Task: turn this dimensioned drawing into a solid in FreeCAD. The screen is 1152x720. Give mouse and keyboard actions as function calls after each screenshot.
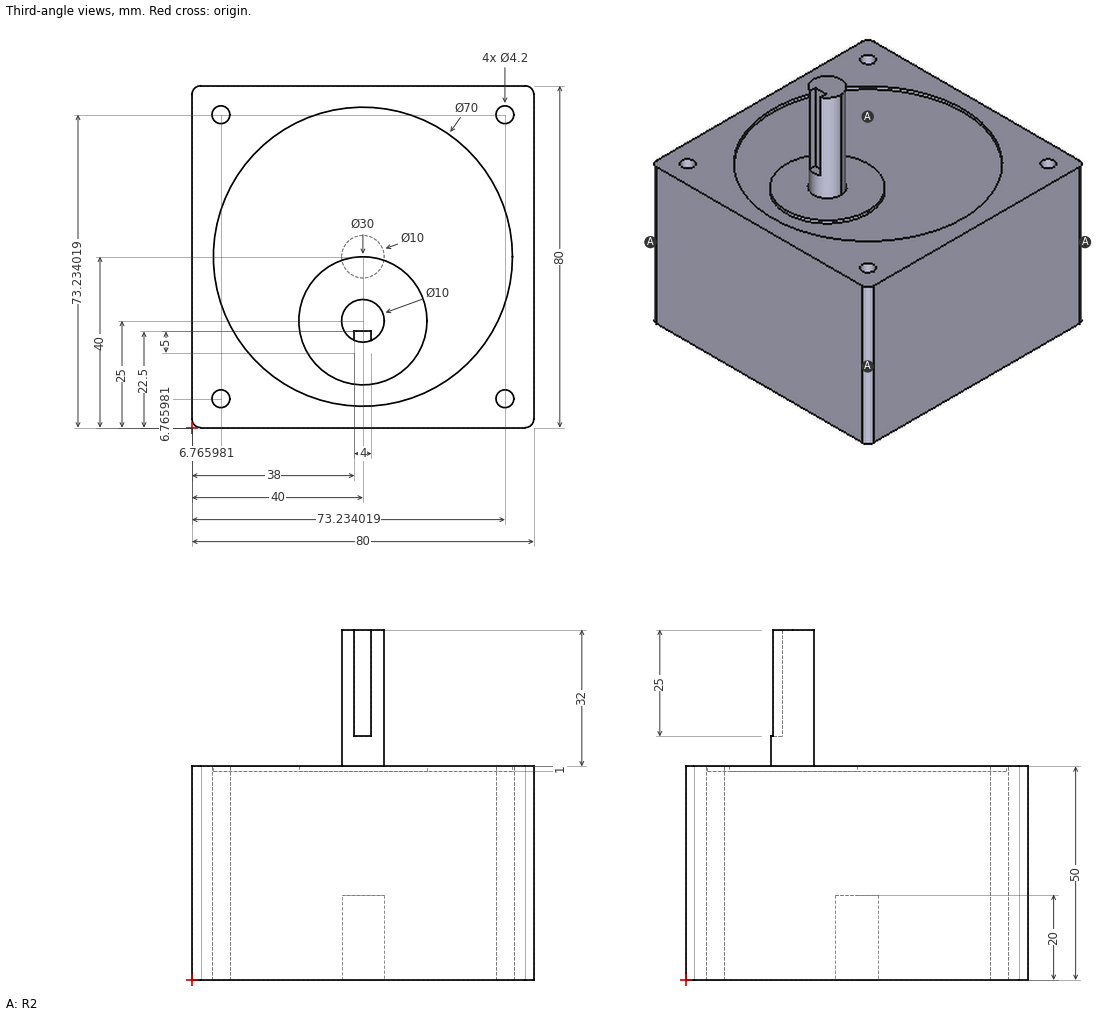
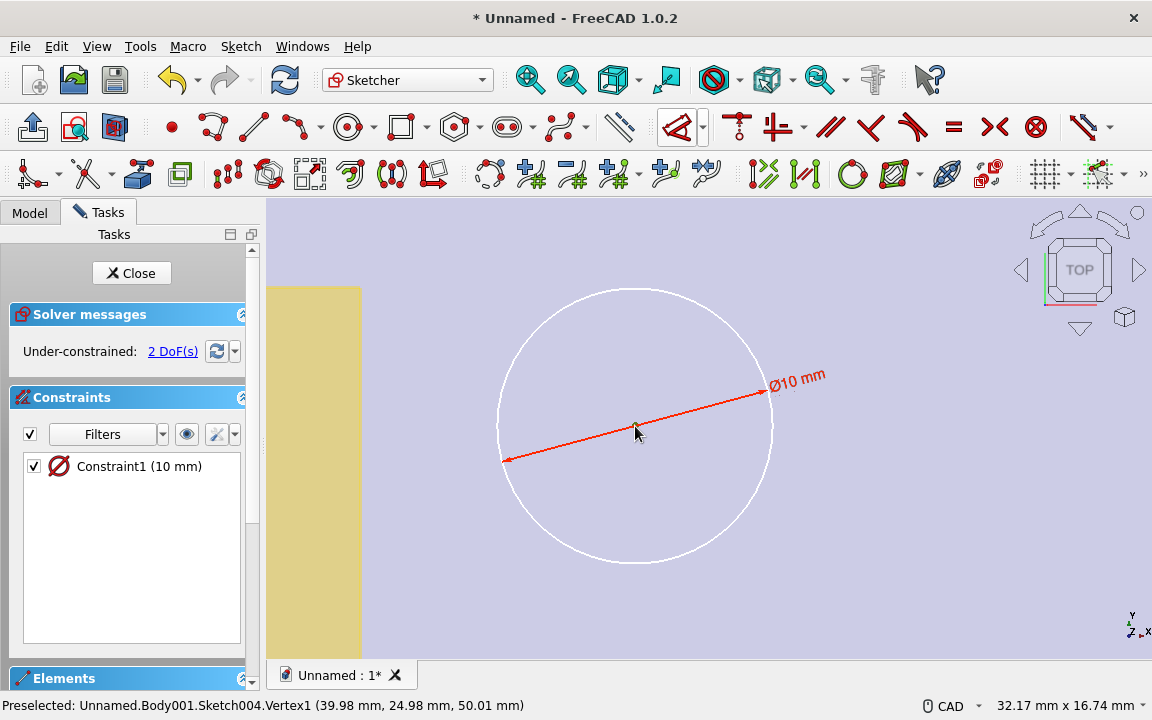
key(l)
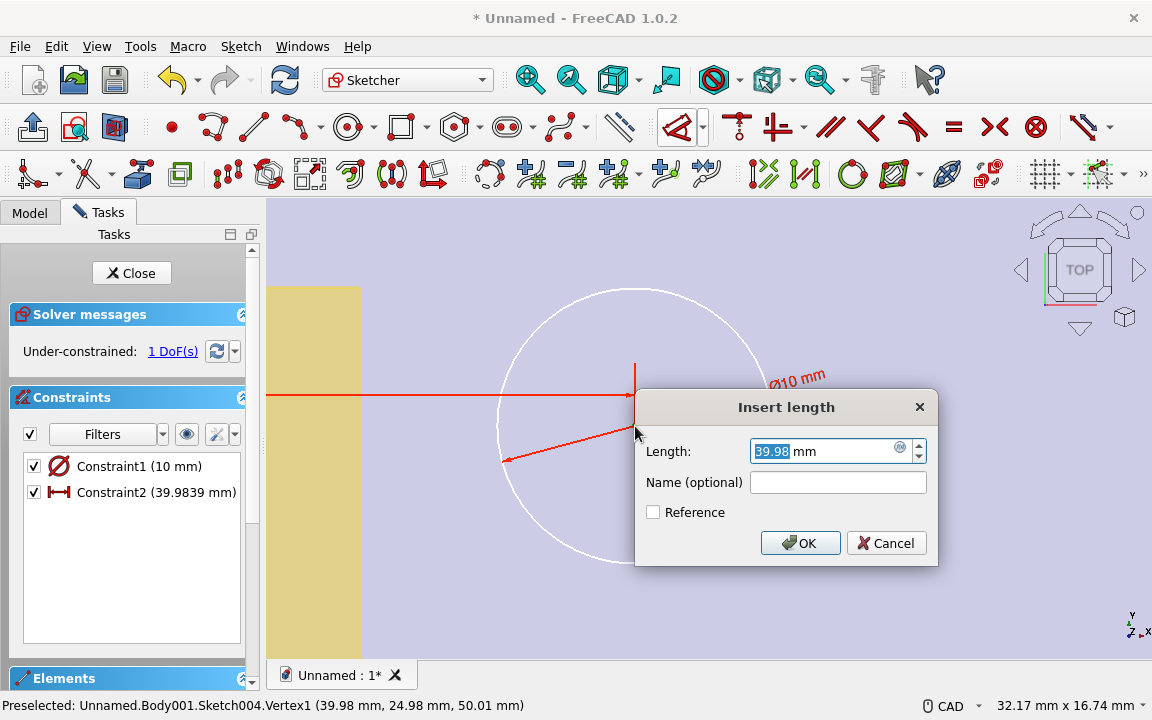
text(40)
key(Return)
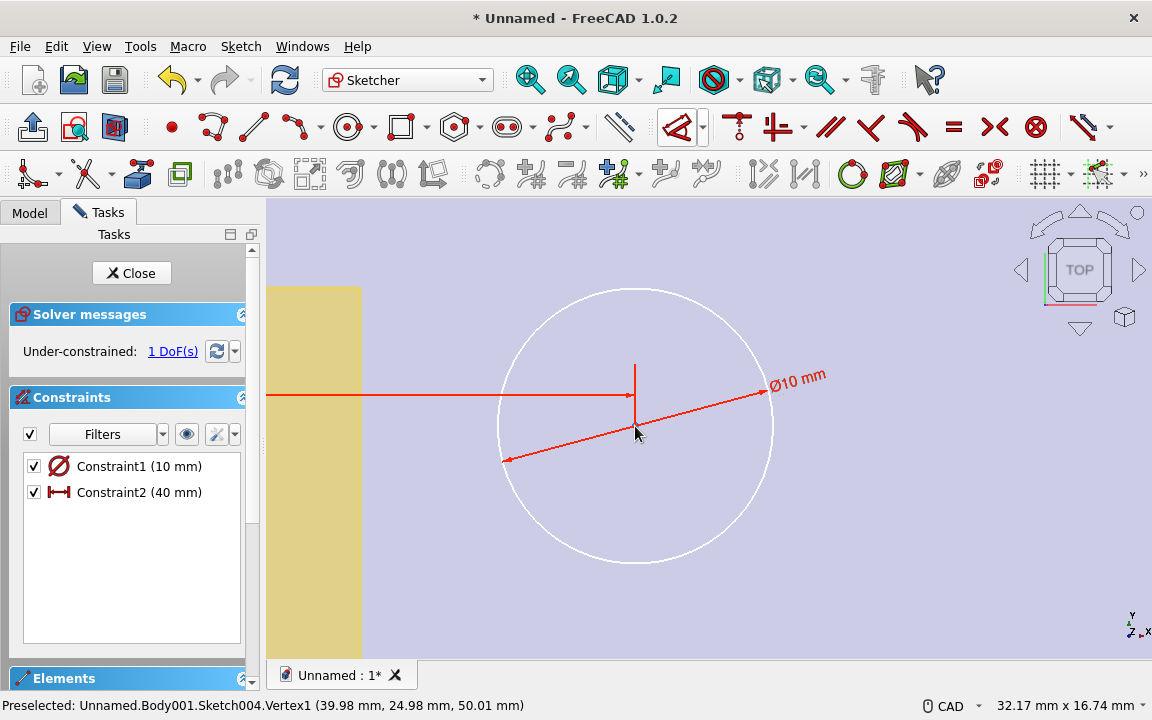
click(635, 426)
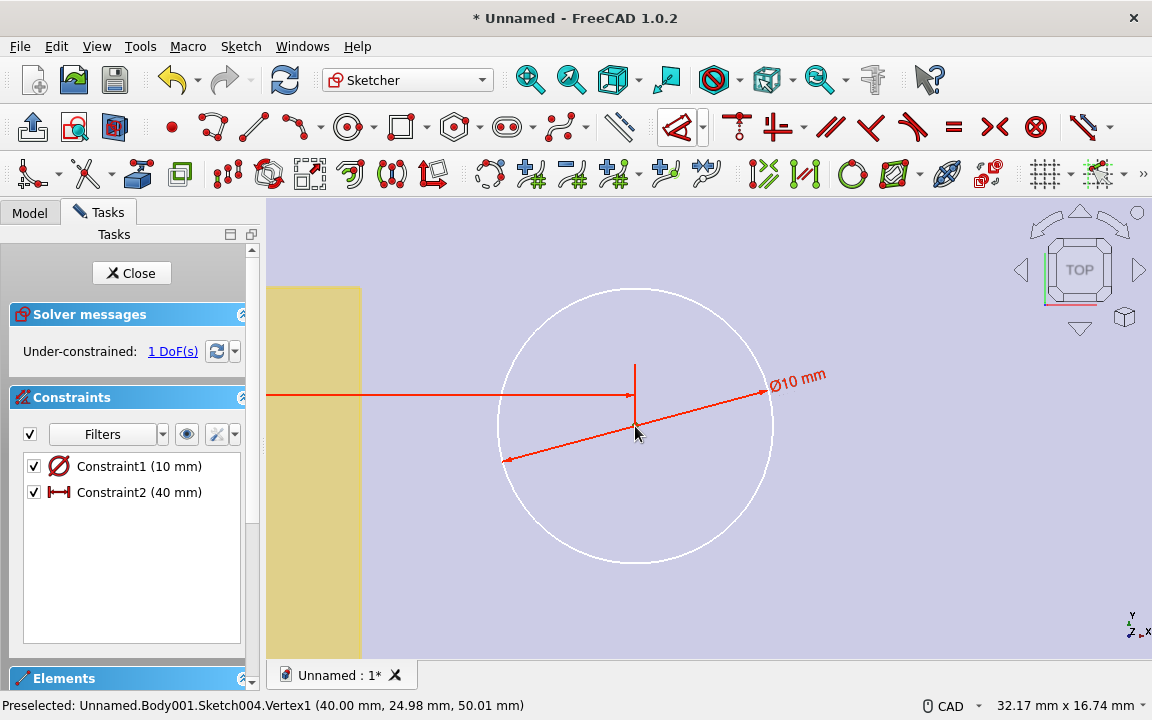
click(702, 128)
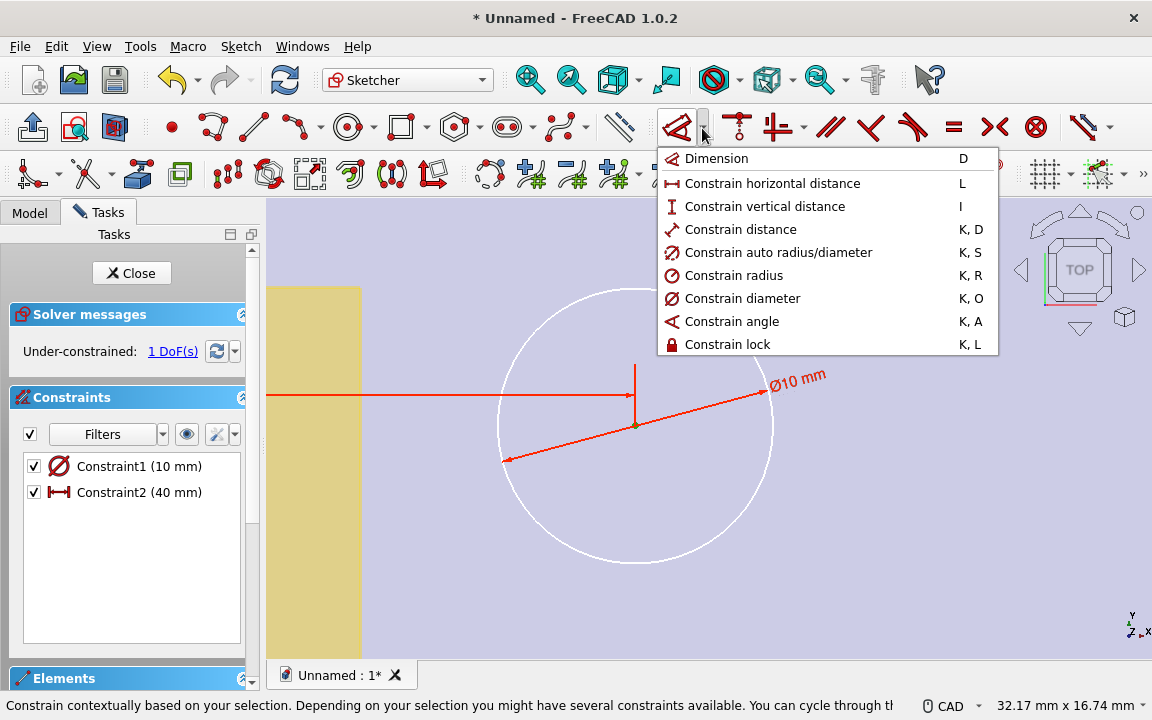
click(828, 206)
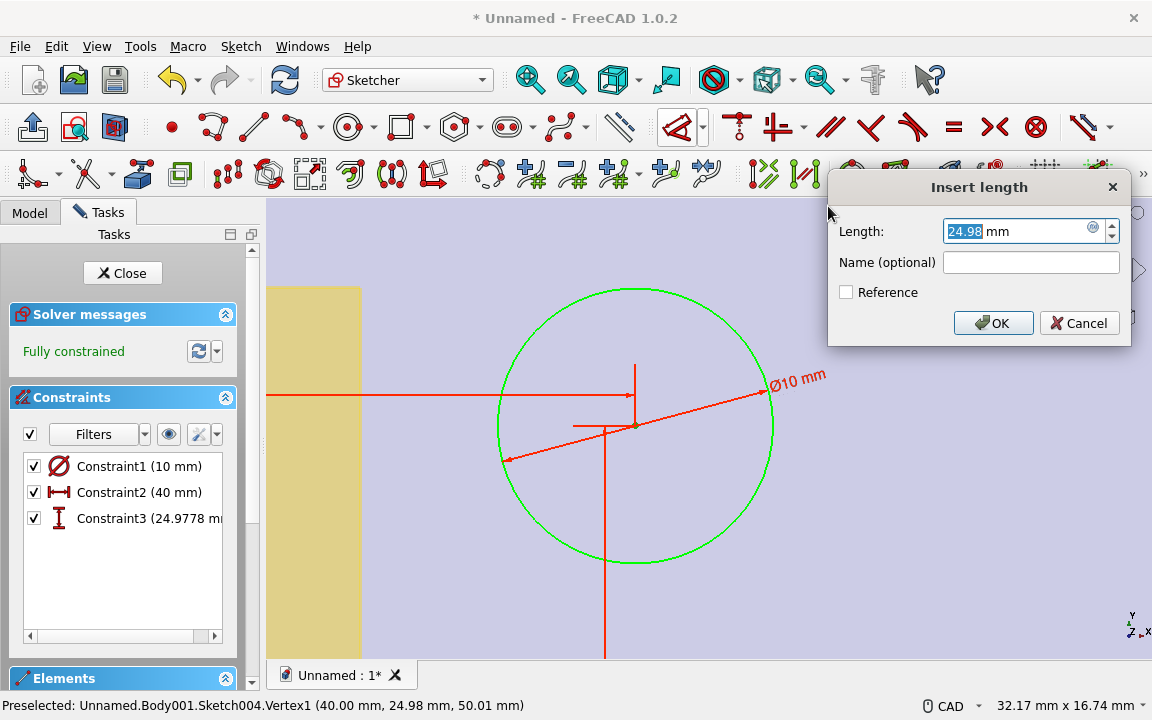
text(25)
key(Return)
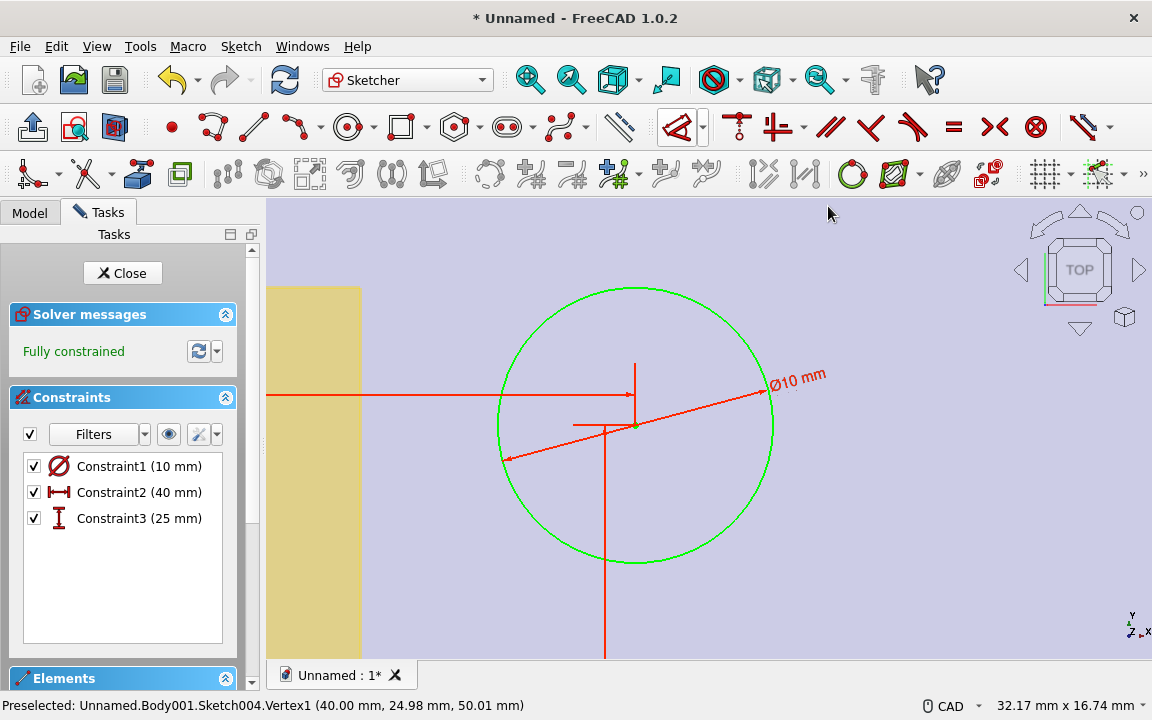
click(123, 273)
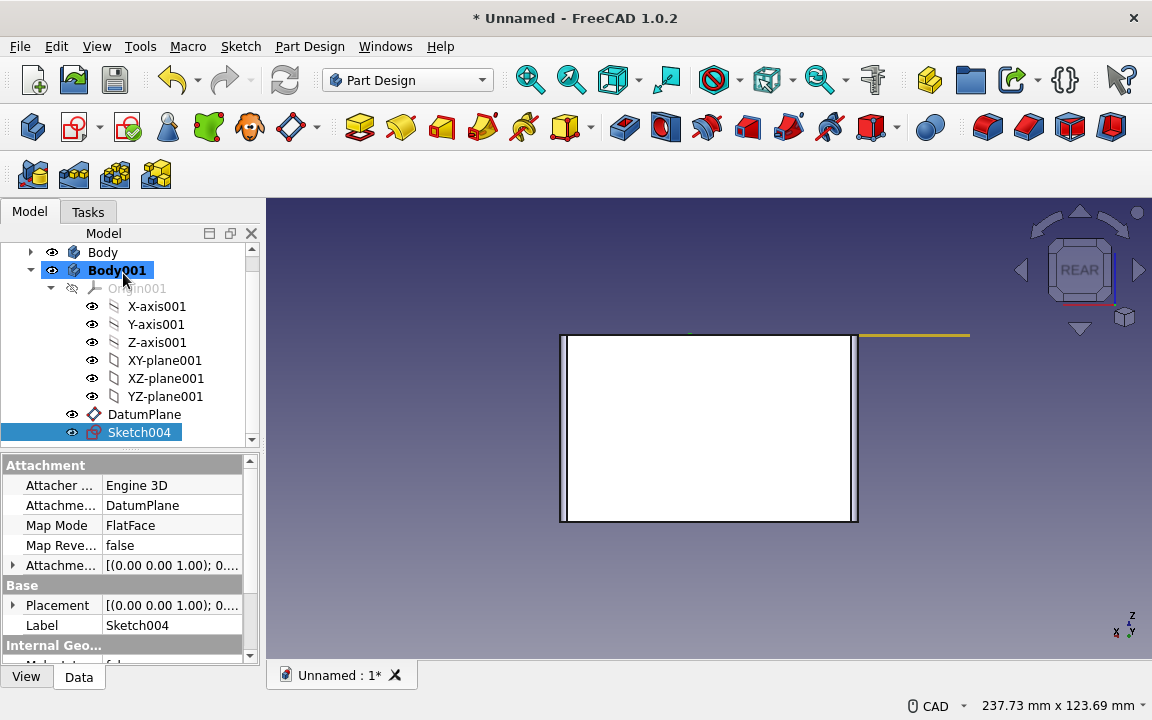
click(360, 128)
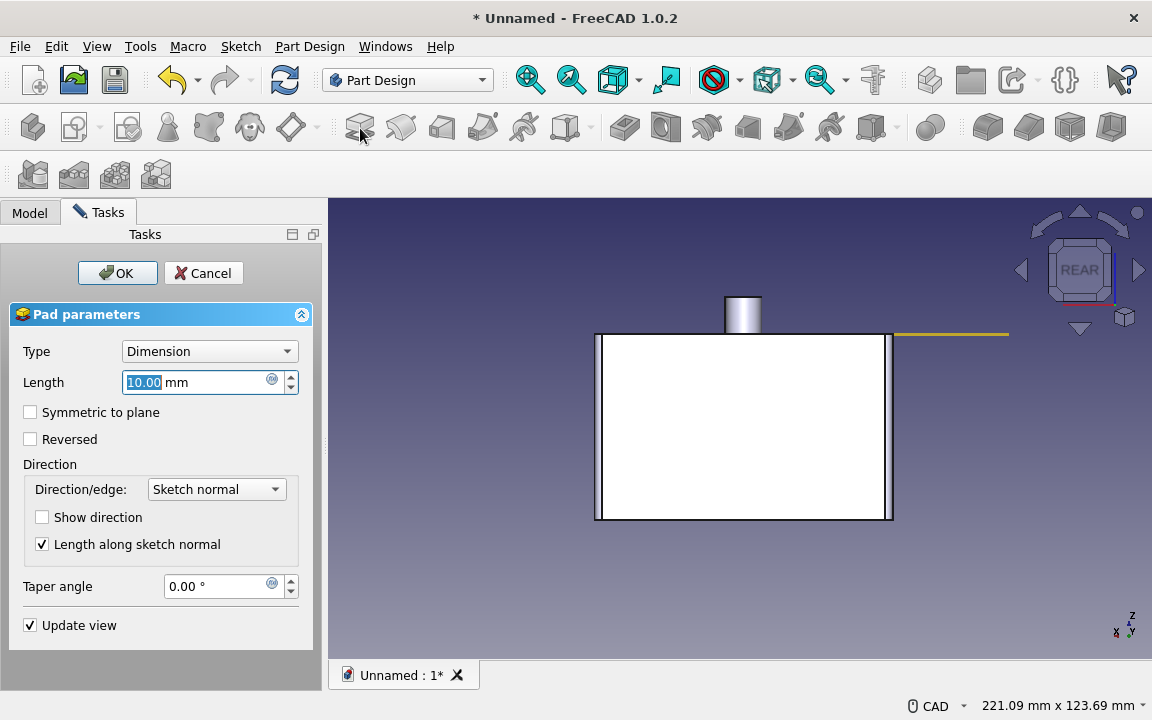
text(32)
key(Tab)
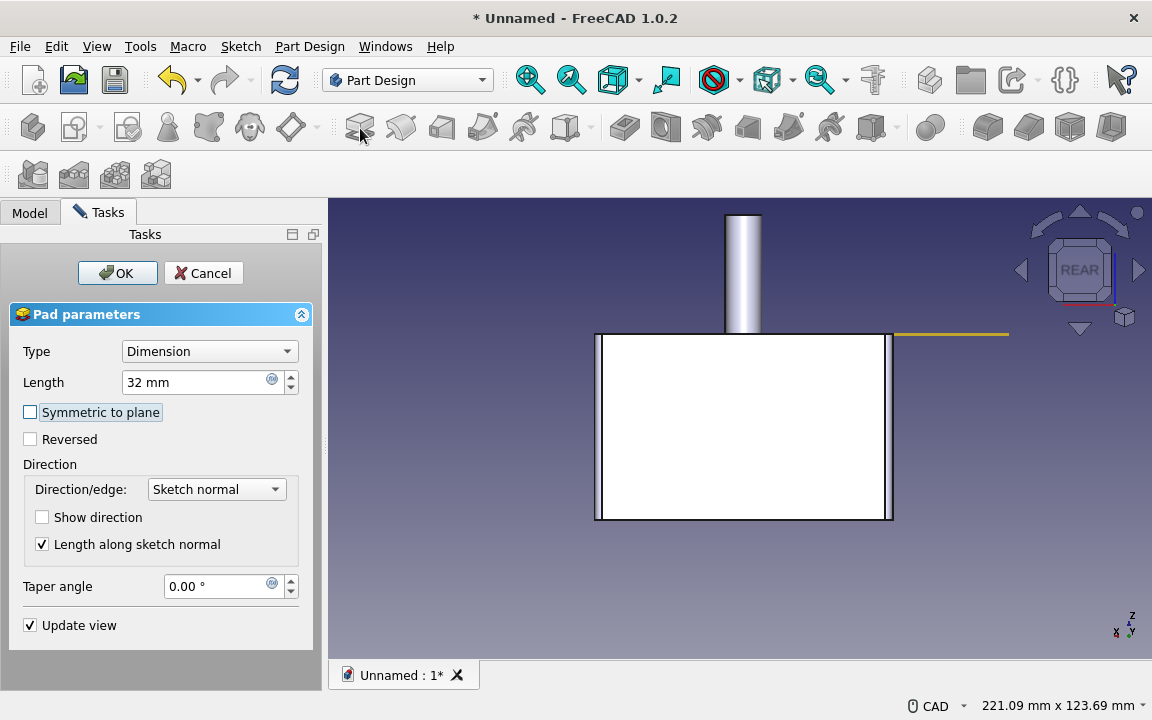
click(118, 273)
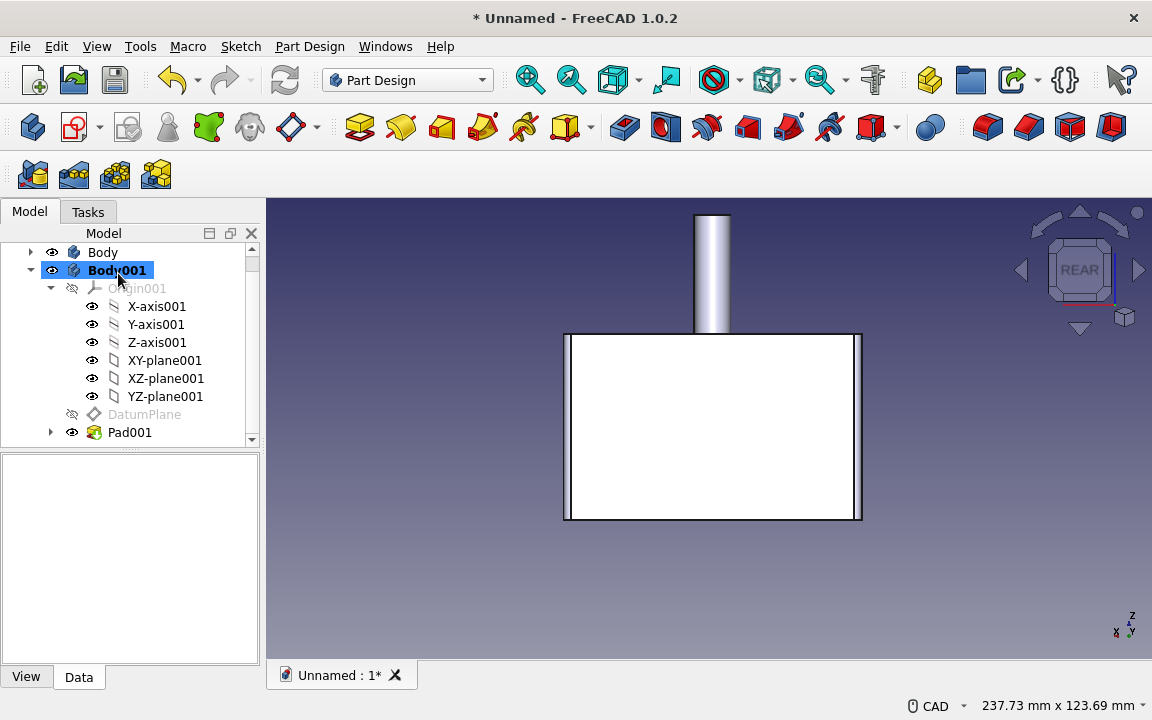
click(531, 80)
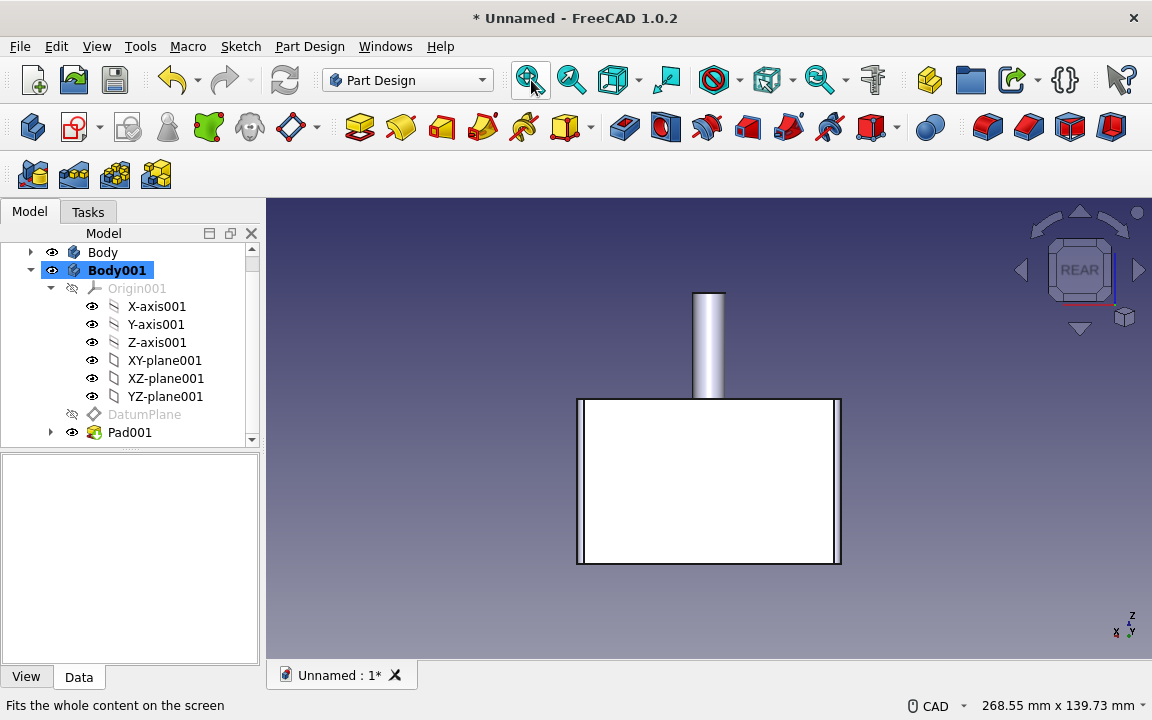
key(0)